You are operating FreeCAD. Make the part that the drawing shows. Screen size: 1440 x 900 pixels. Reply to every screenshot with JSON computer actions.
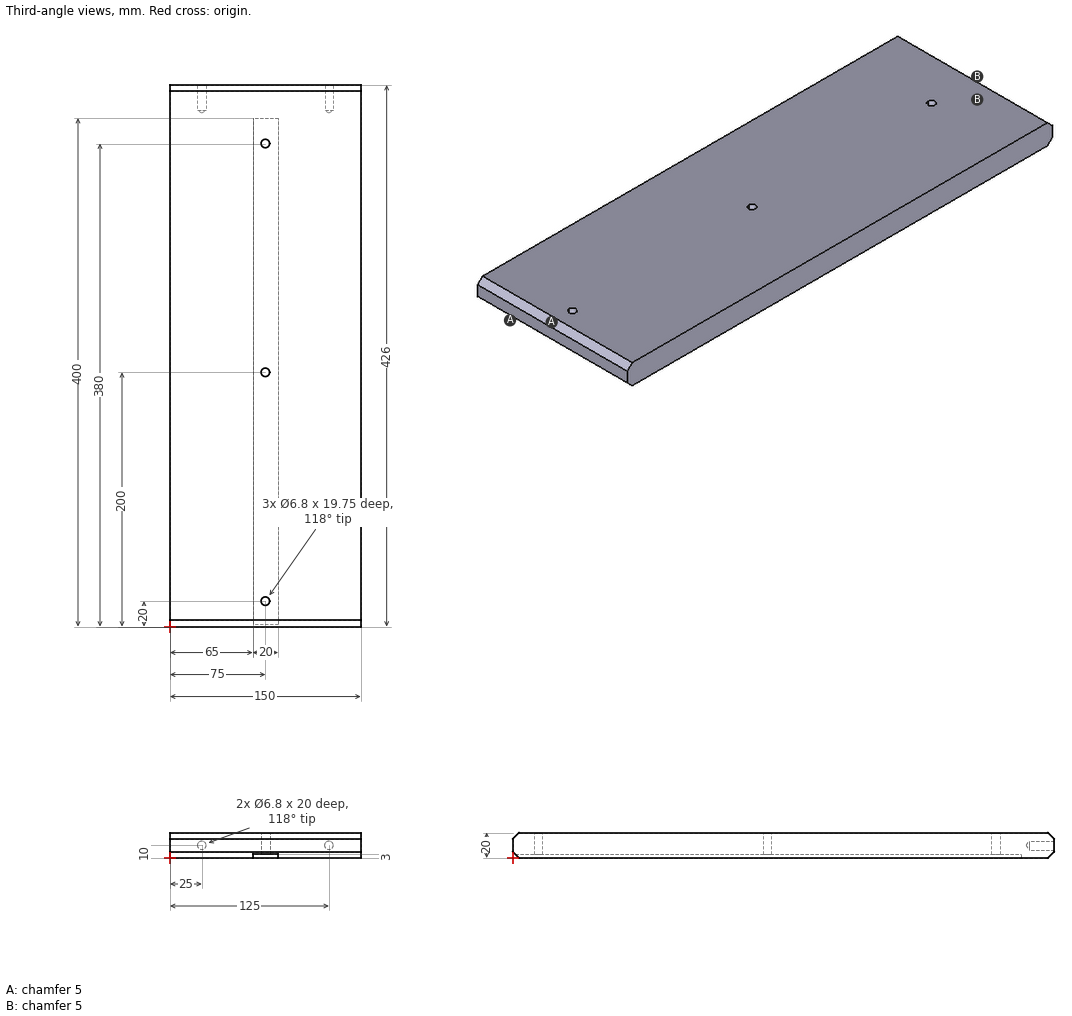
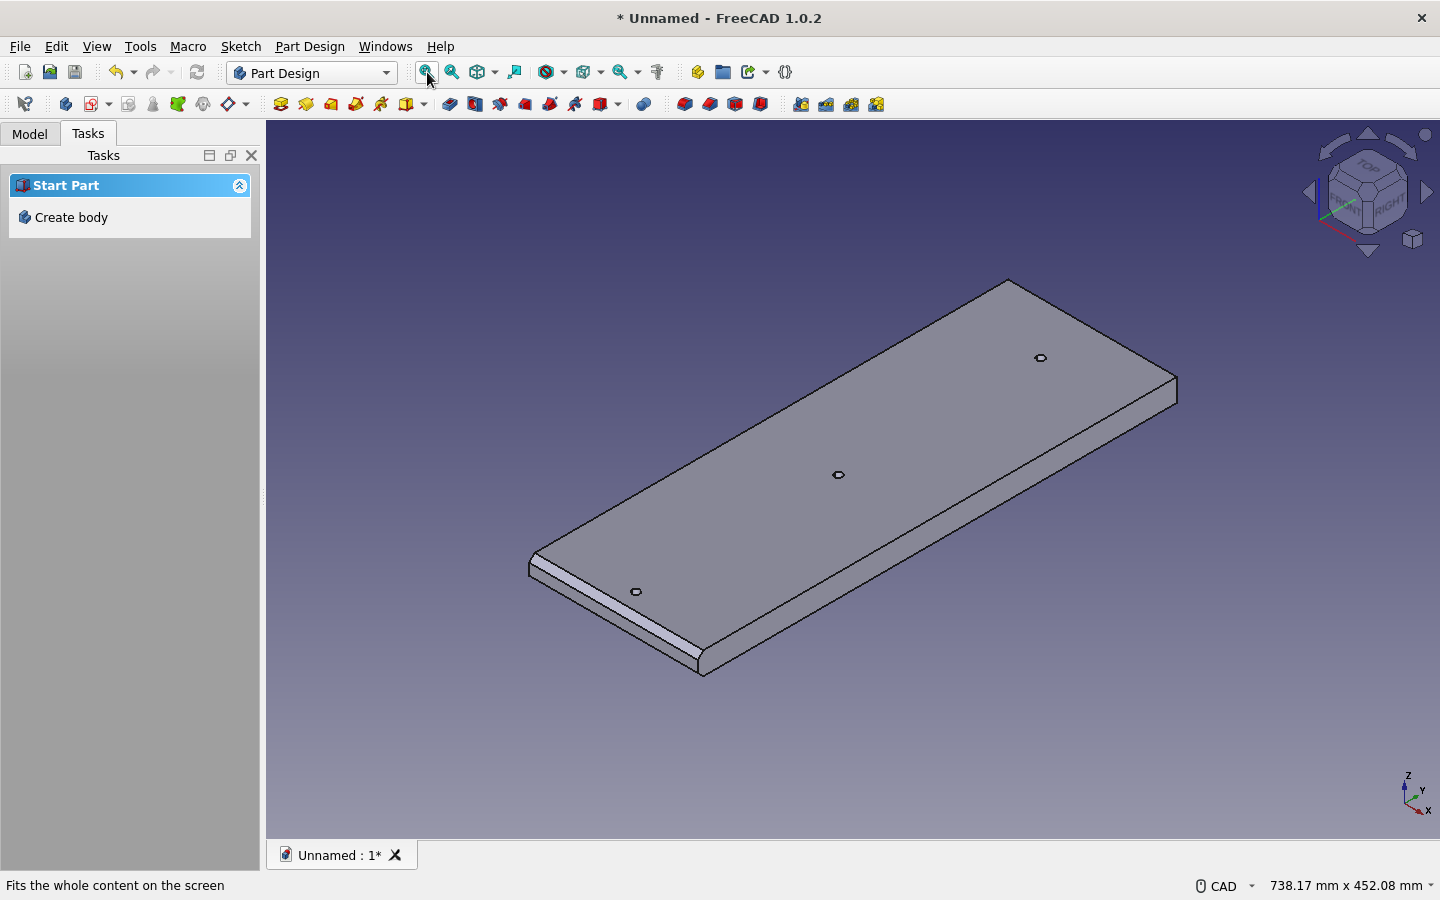
{"action": "key", "text": "2"}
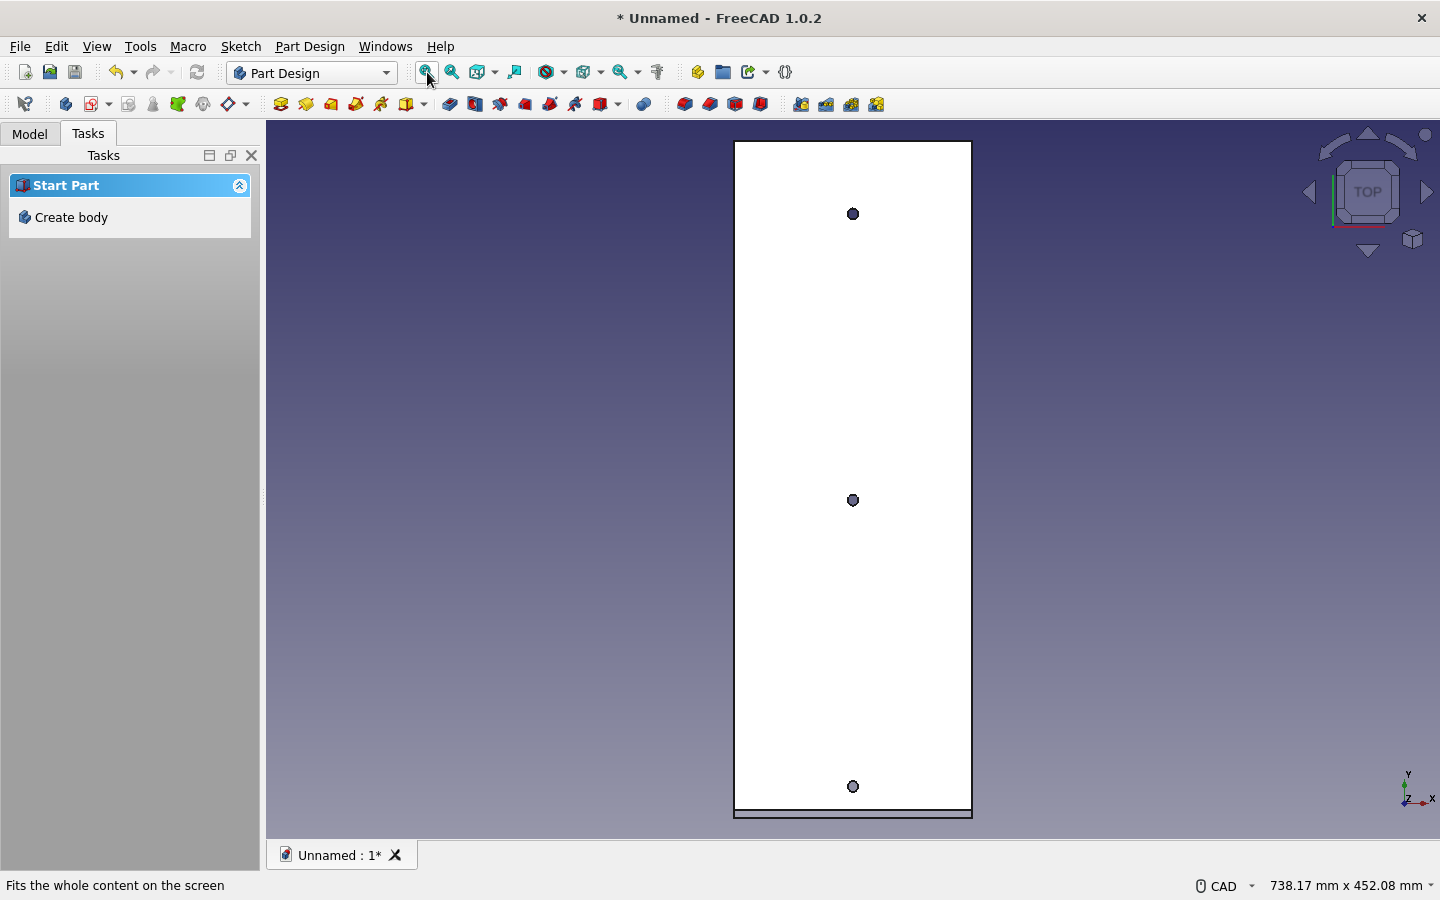
{"action": "key", "text": "1"}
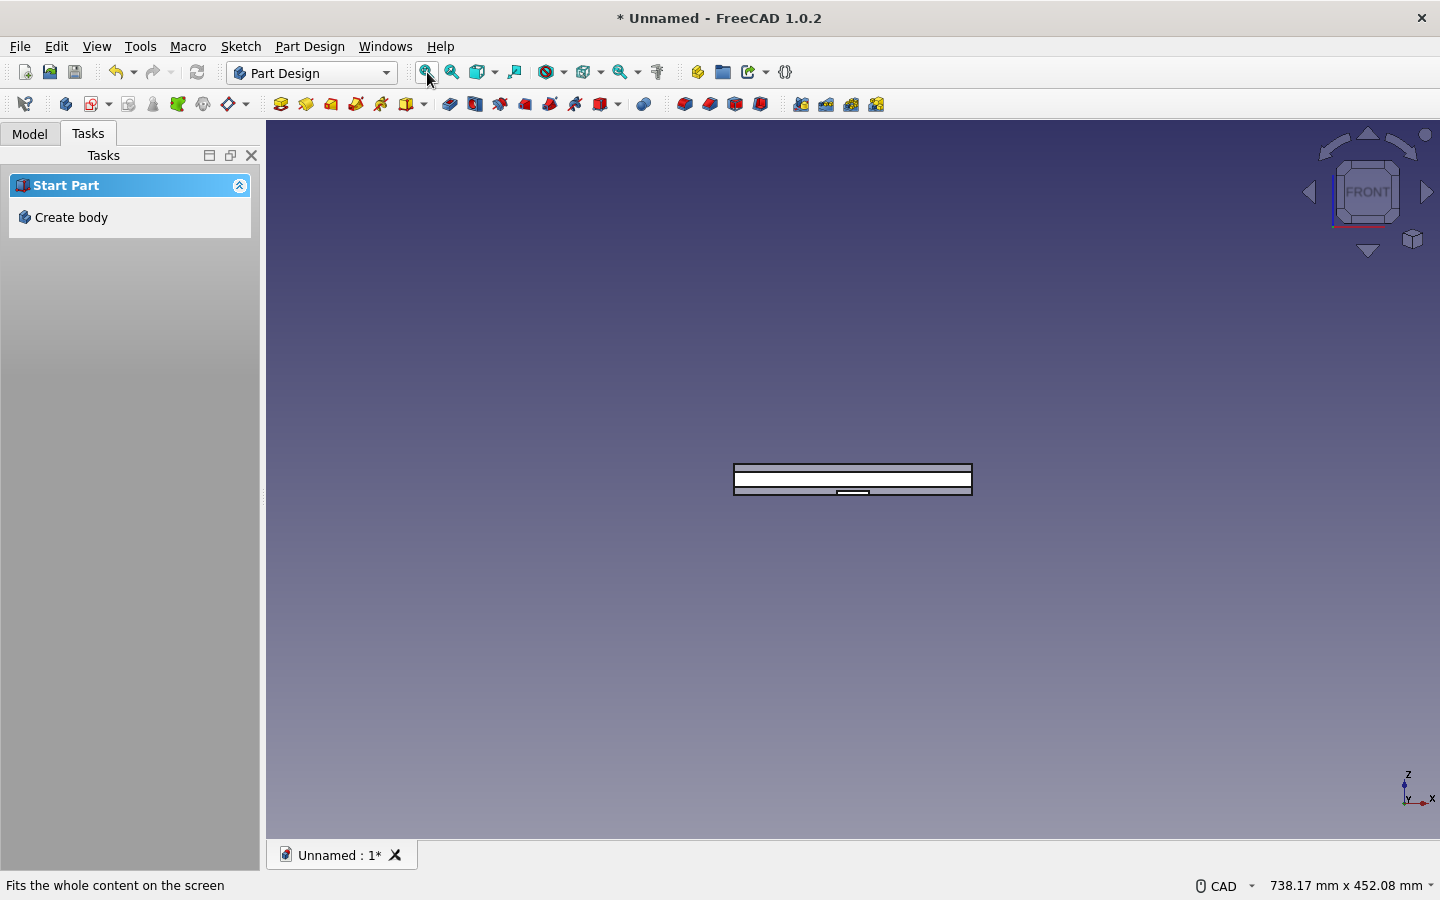
{"action": "left_click", "coordinate": [427, 72]}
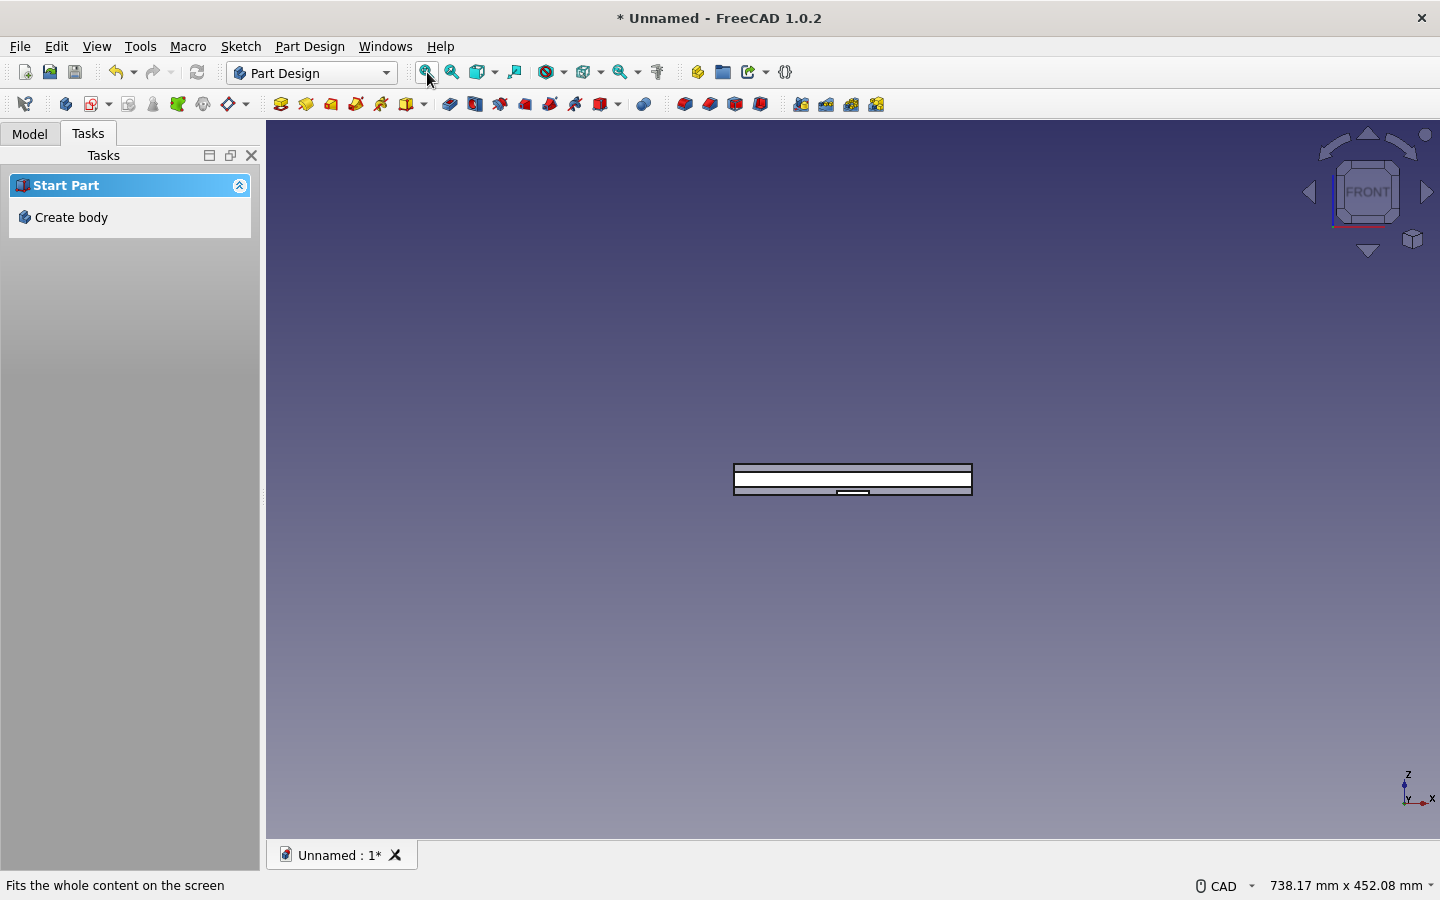
{"action": "key", "text": "3"}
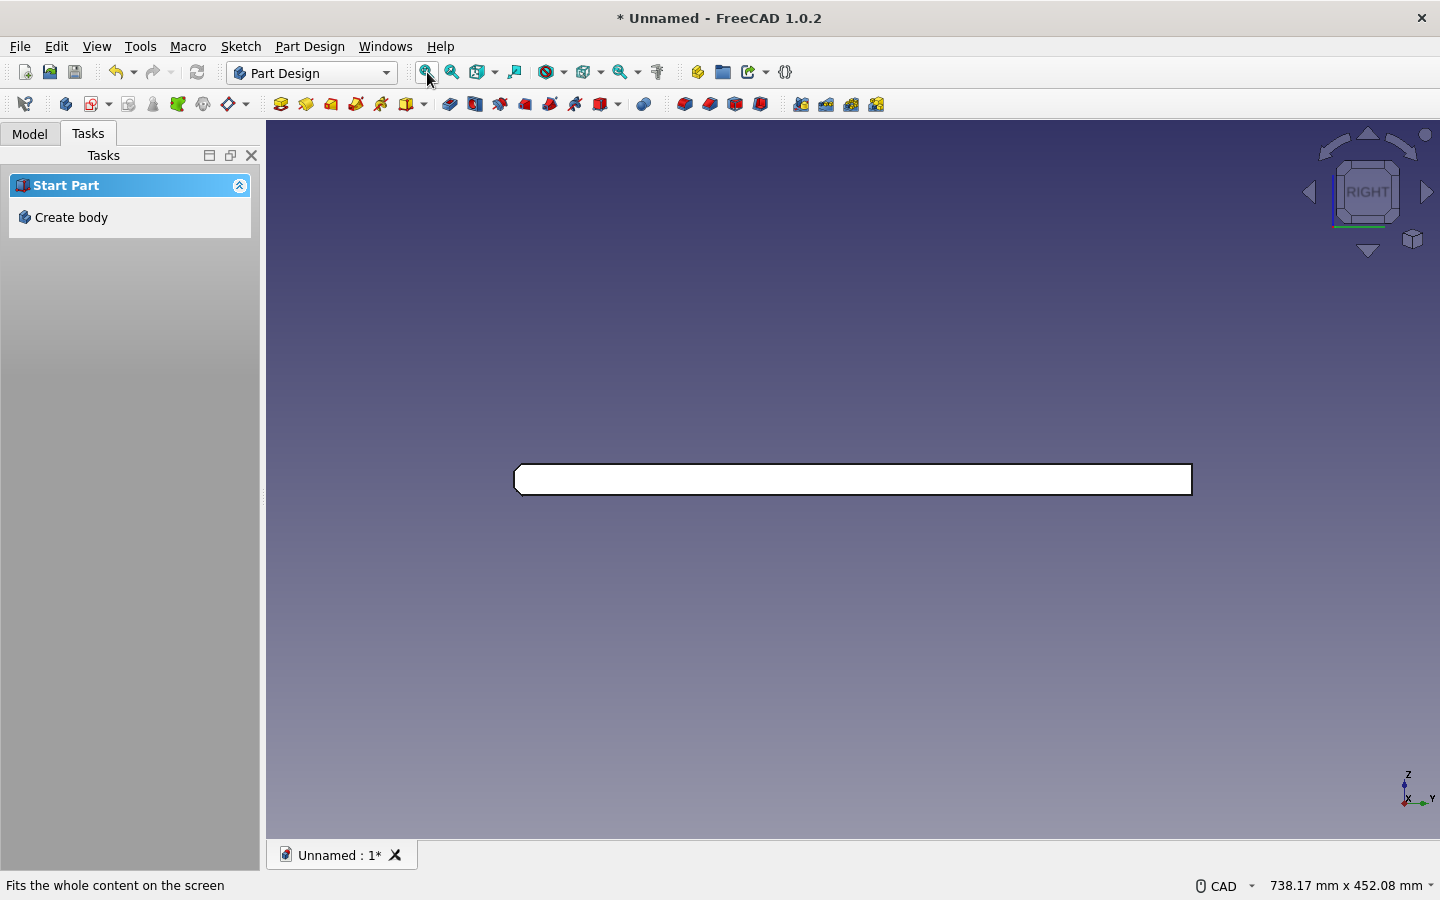
{"action": "key", "text": "5"}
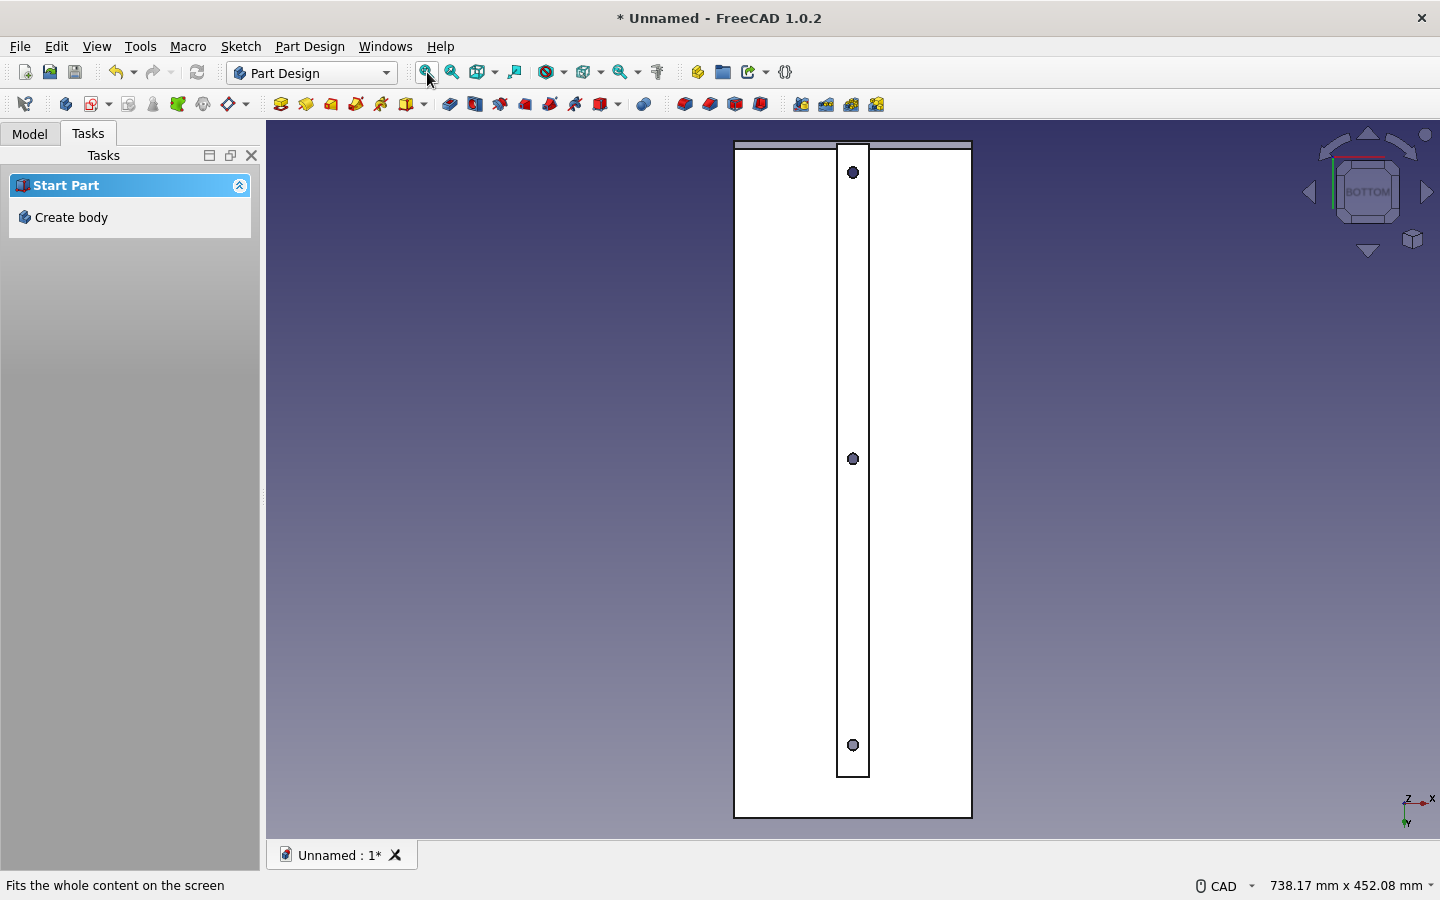
{"action": "key", "text": "4"}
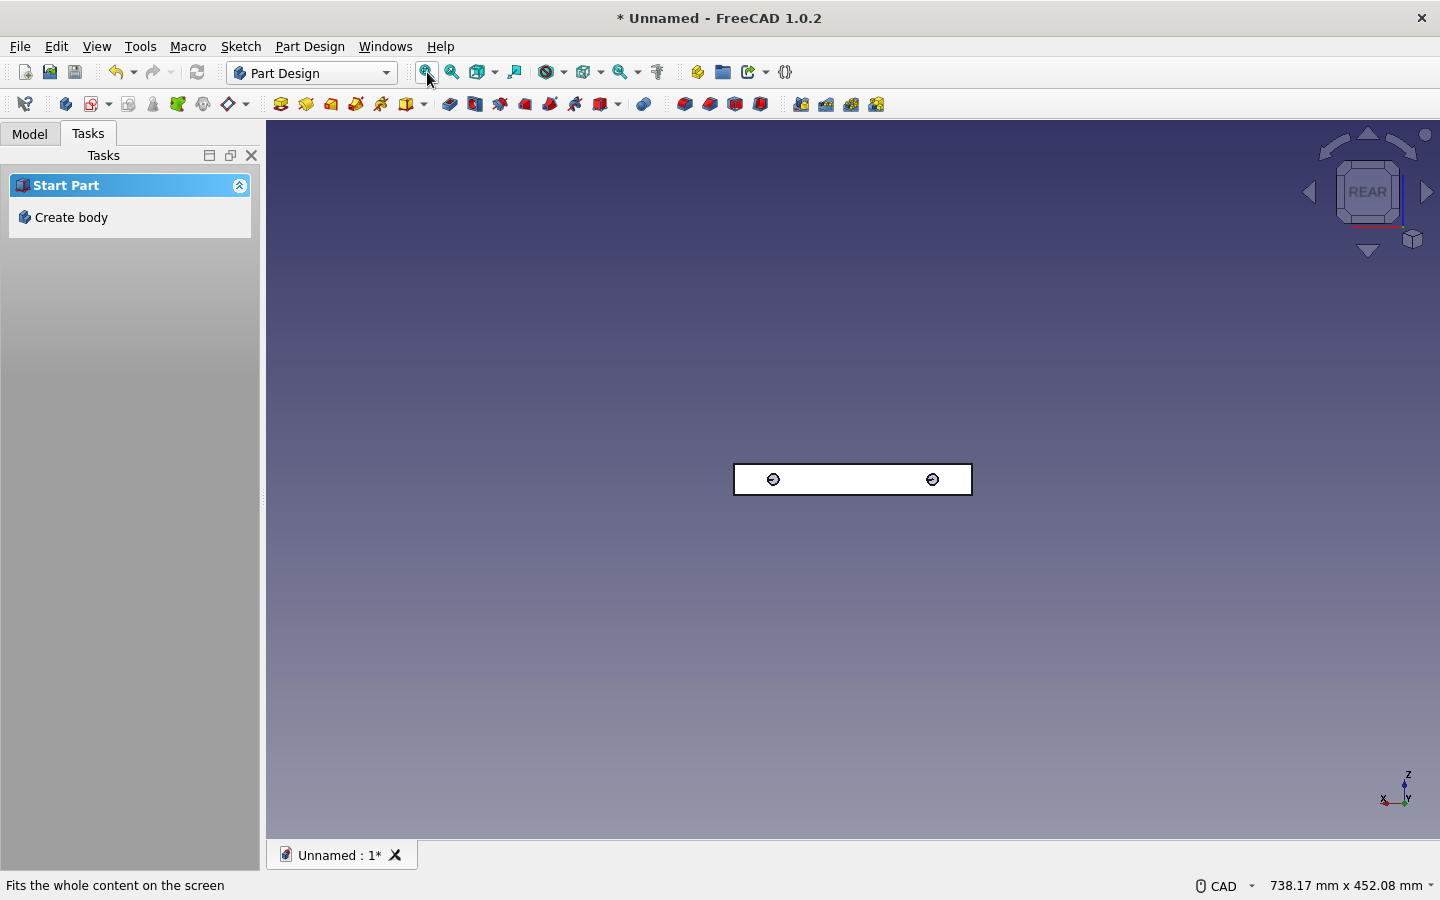
{"action": "left_click", "coordinate": [427, 72]}